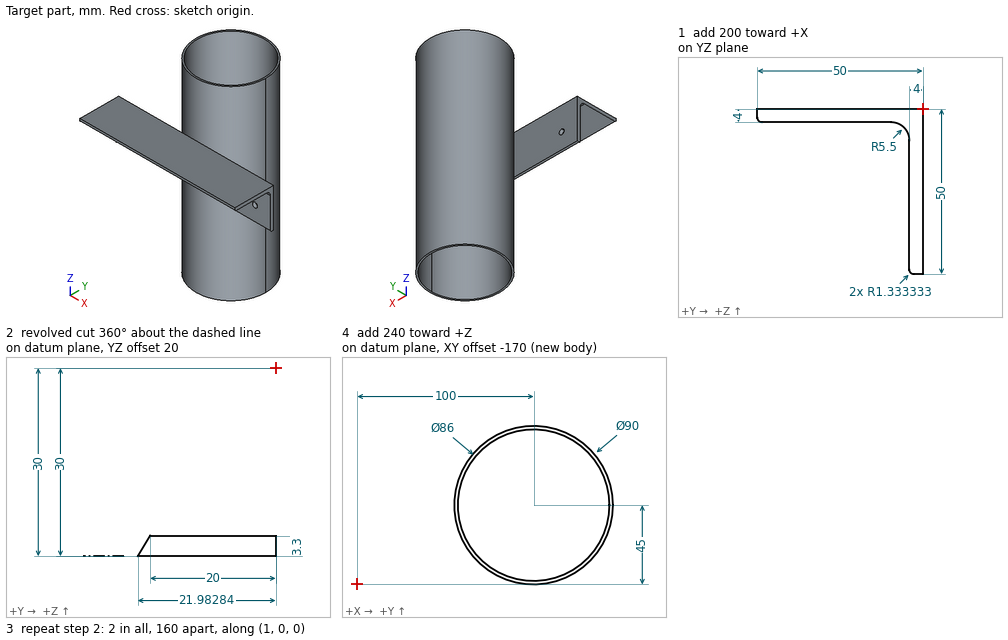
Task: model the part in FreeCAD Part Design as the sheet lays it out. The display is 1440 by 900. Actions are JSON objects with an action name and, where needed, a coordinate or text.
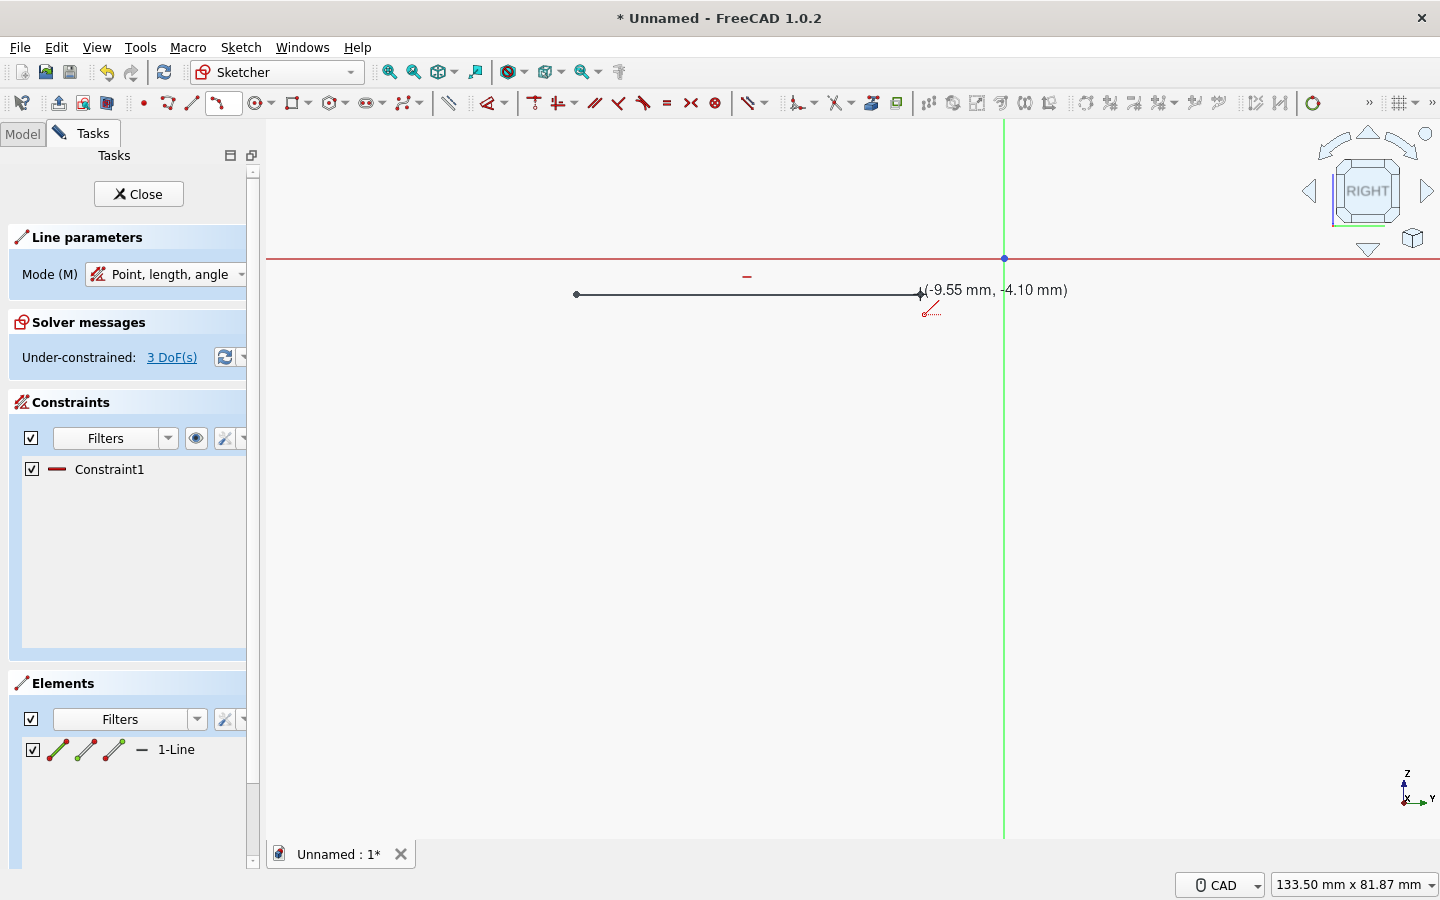
{"action": "left_click", "coordinate": [969, 343]}
{"action": "left_click", "coordinate": [969, 687]}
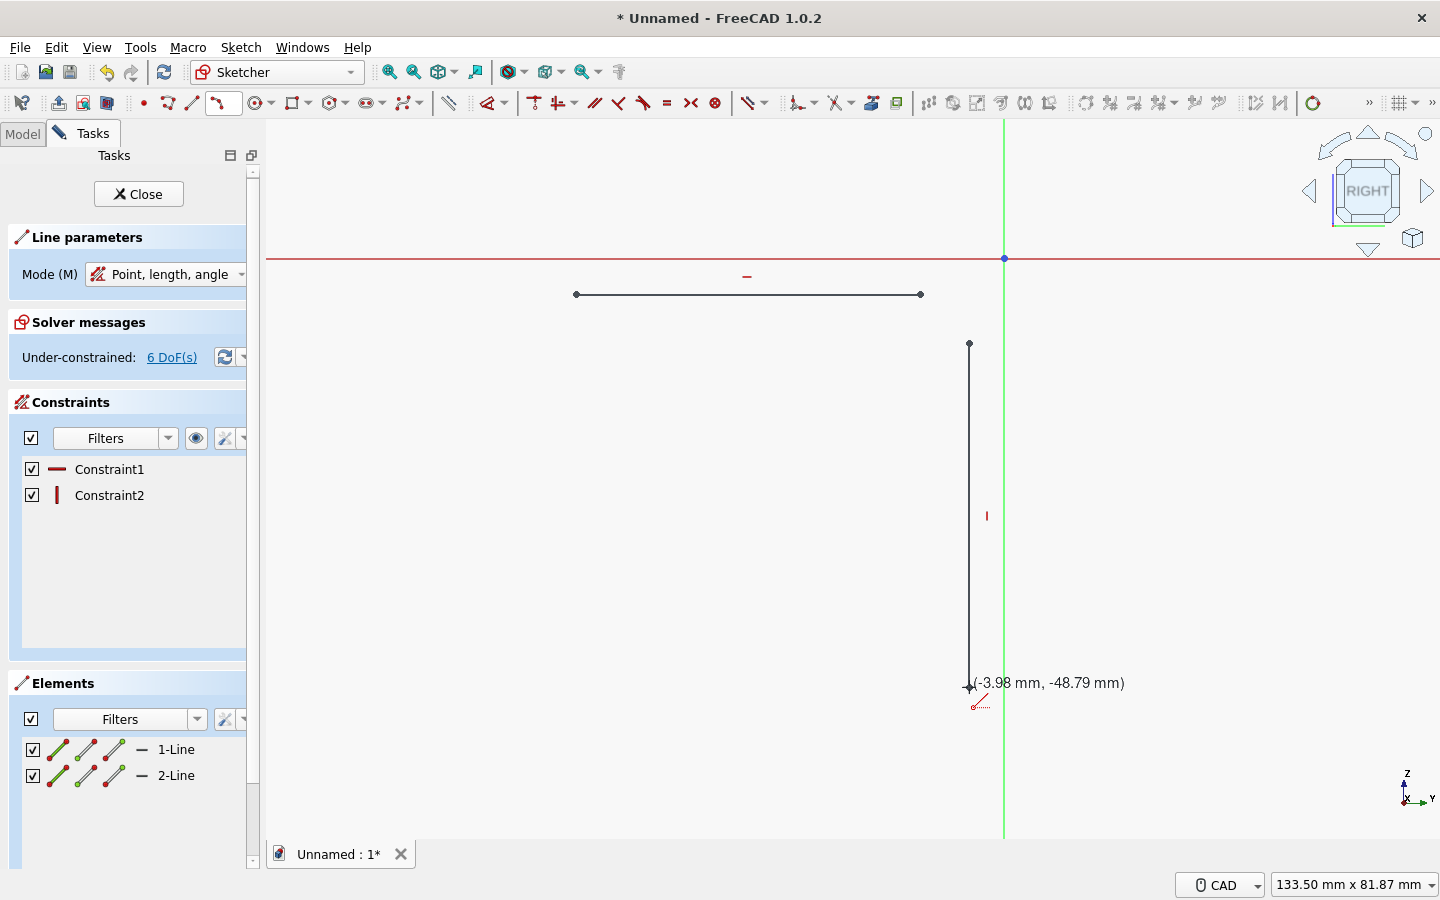
{"action": "left_click", "coordinate": [168, 104]}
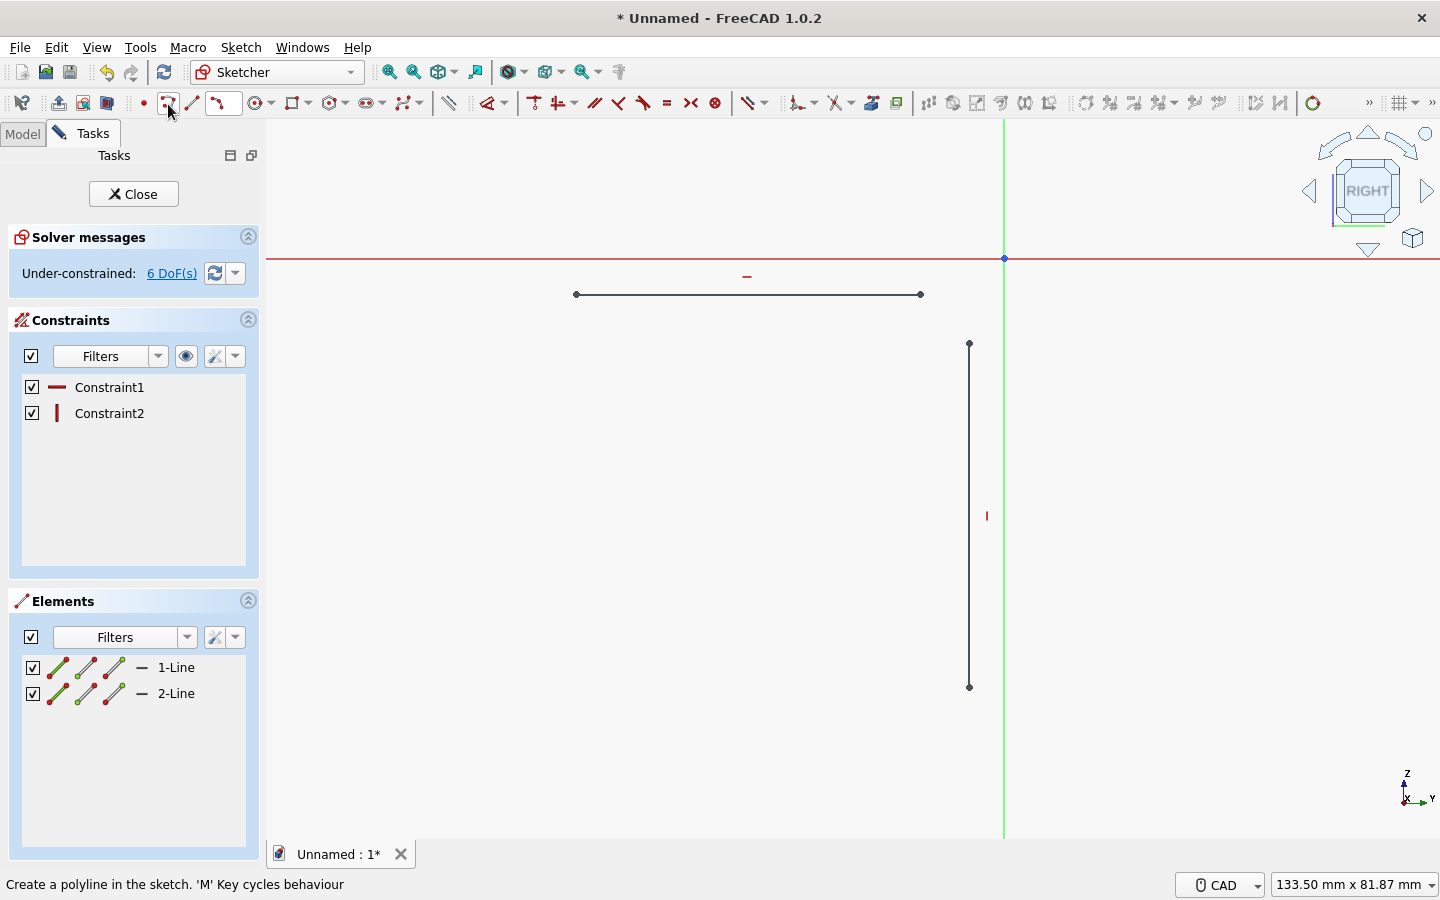
{"action": "left_click", "coordinate": [981, 699]}
{"action": "left_click", "coordinate": [1004, 699]}
{"action": "left_click", "coordinate": [1004, 259]}
{"action": "left_click", "coordinate": [564, 268]}
{"action": "left_click", "coordinate": [564, 282]}
{"action": "right_click", "coordinate": [564, 282]}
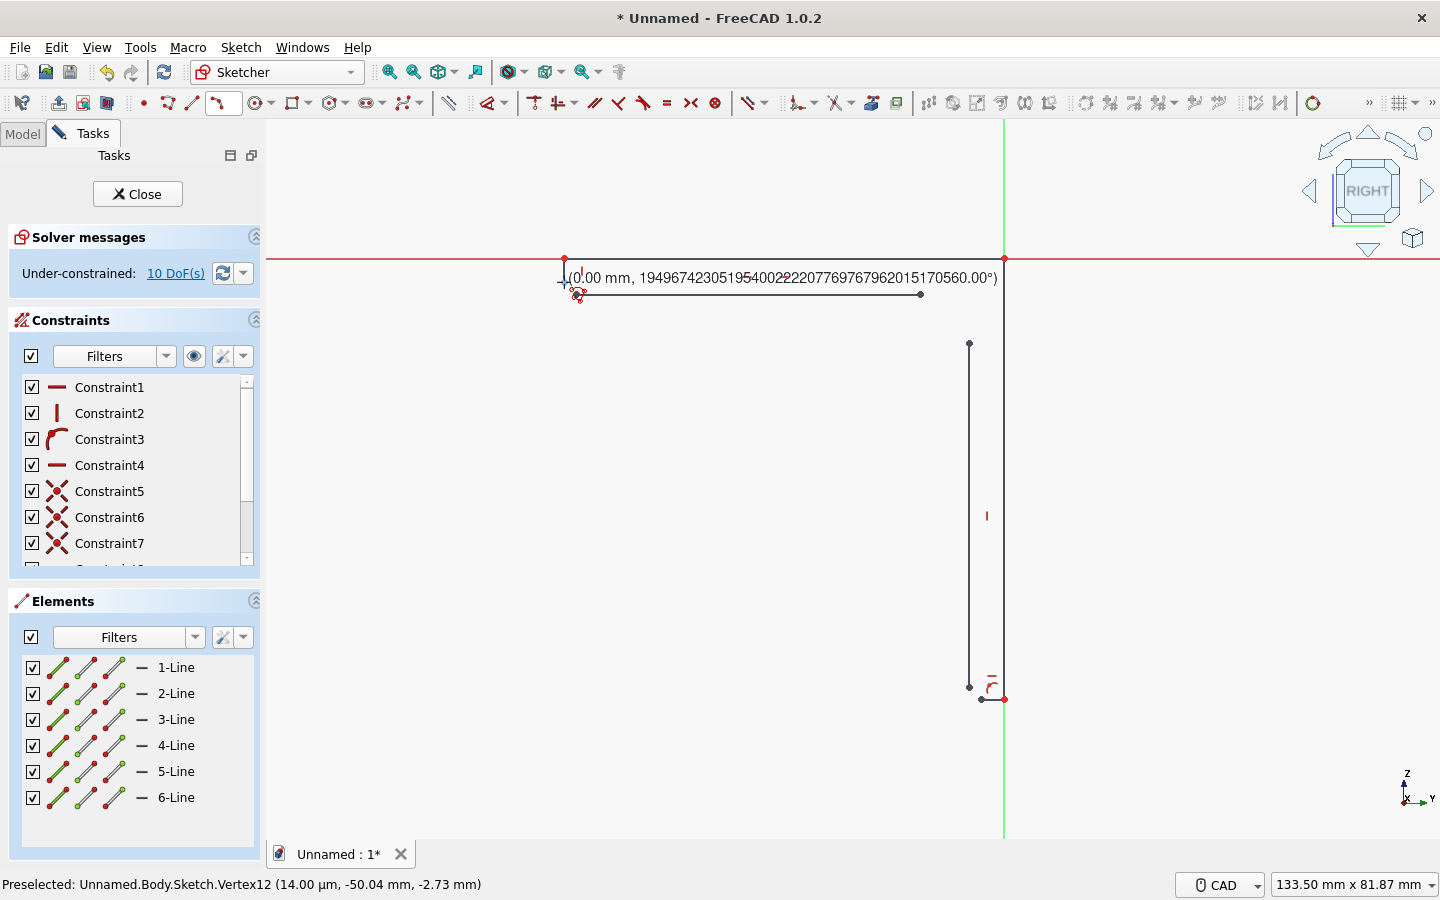
{"action": "left_click", "coordinate": [218, 104]}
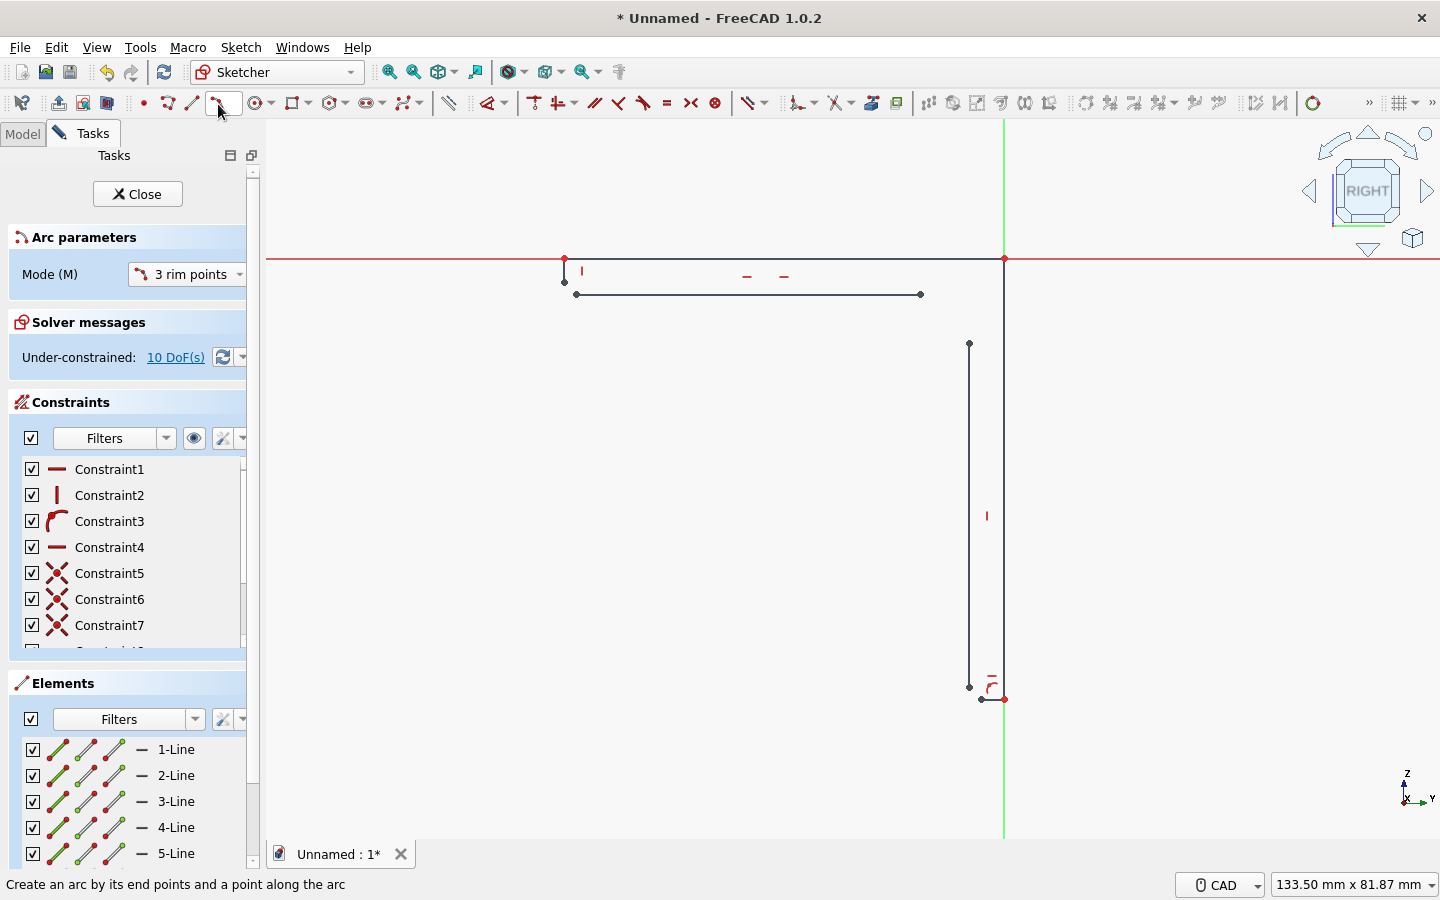
{"action": "left_click", "coordinate": [920, 295]}
{"action": "left_click", "coordinate": [969, 344]}
{"action": "left_click", "coordinate": [955, 308]}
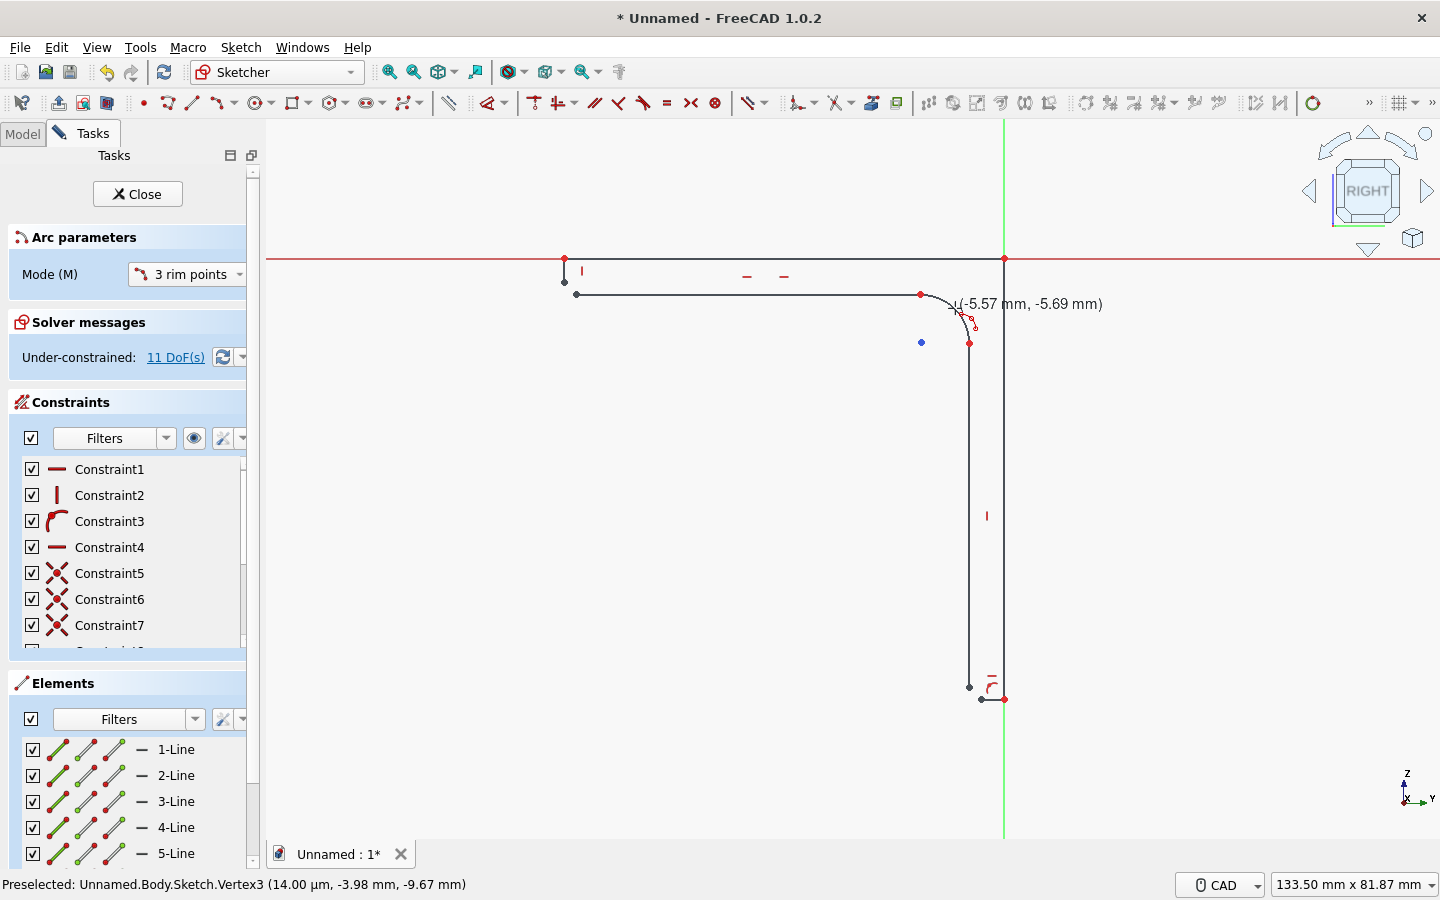
{"action": "left_click", "coordinate": [969, 688]}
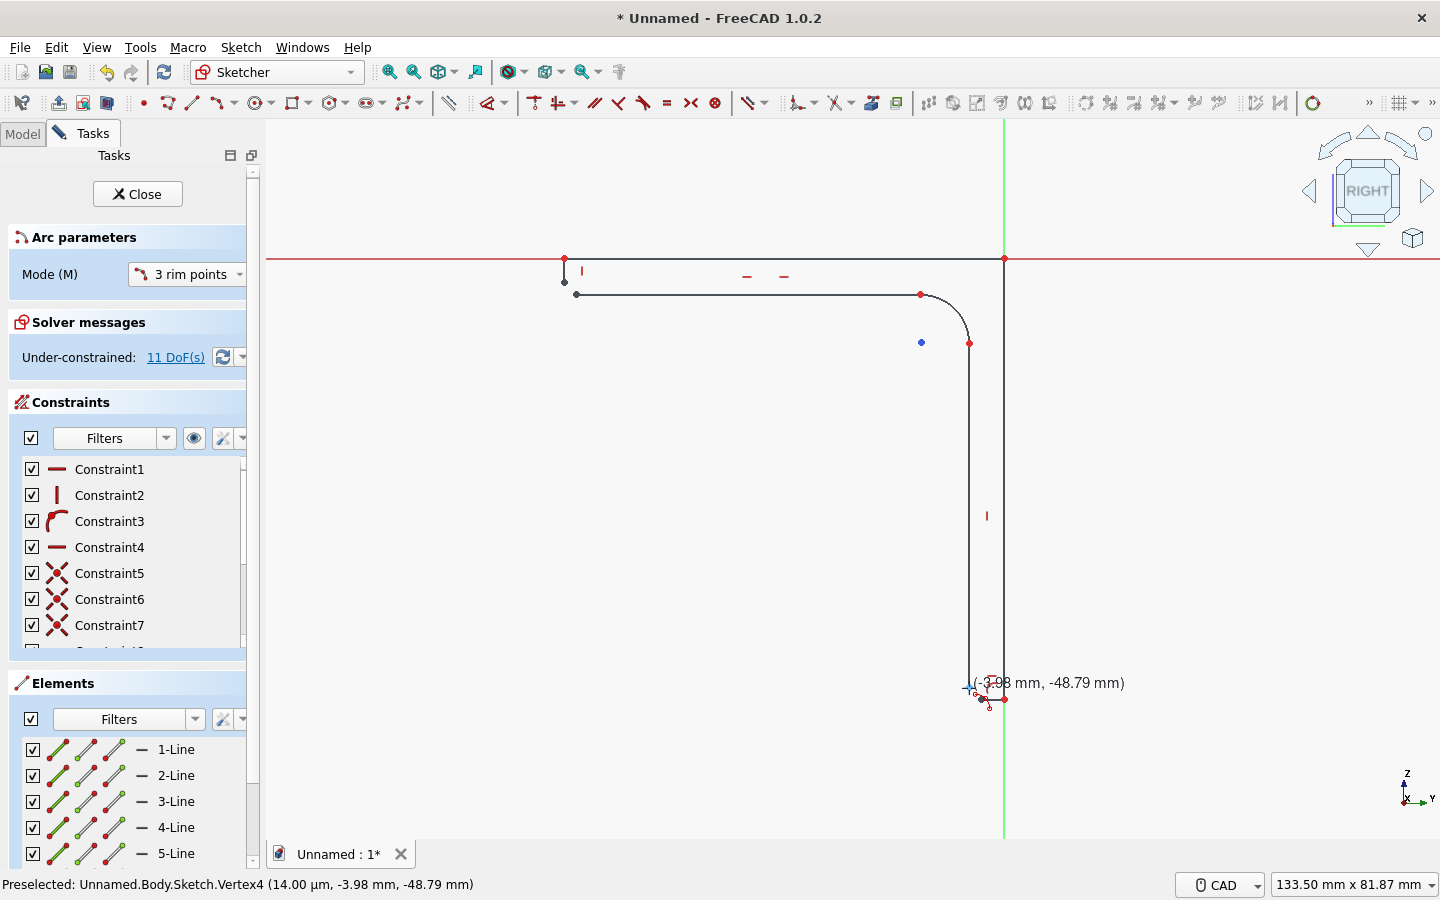
{"action": "scroll", "coordinate": [981, 699], "scroll_direction": "up", "scroll_amount": 2}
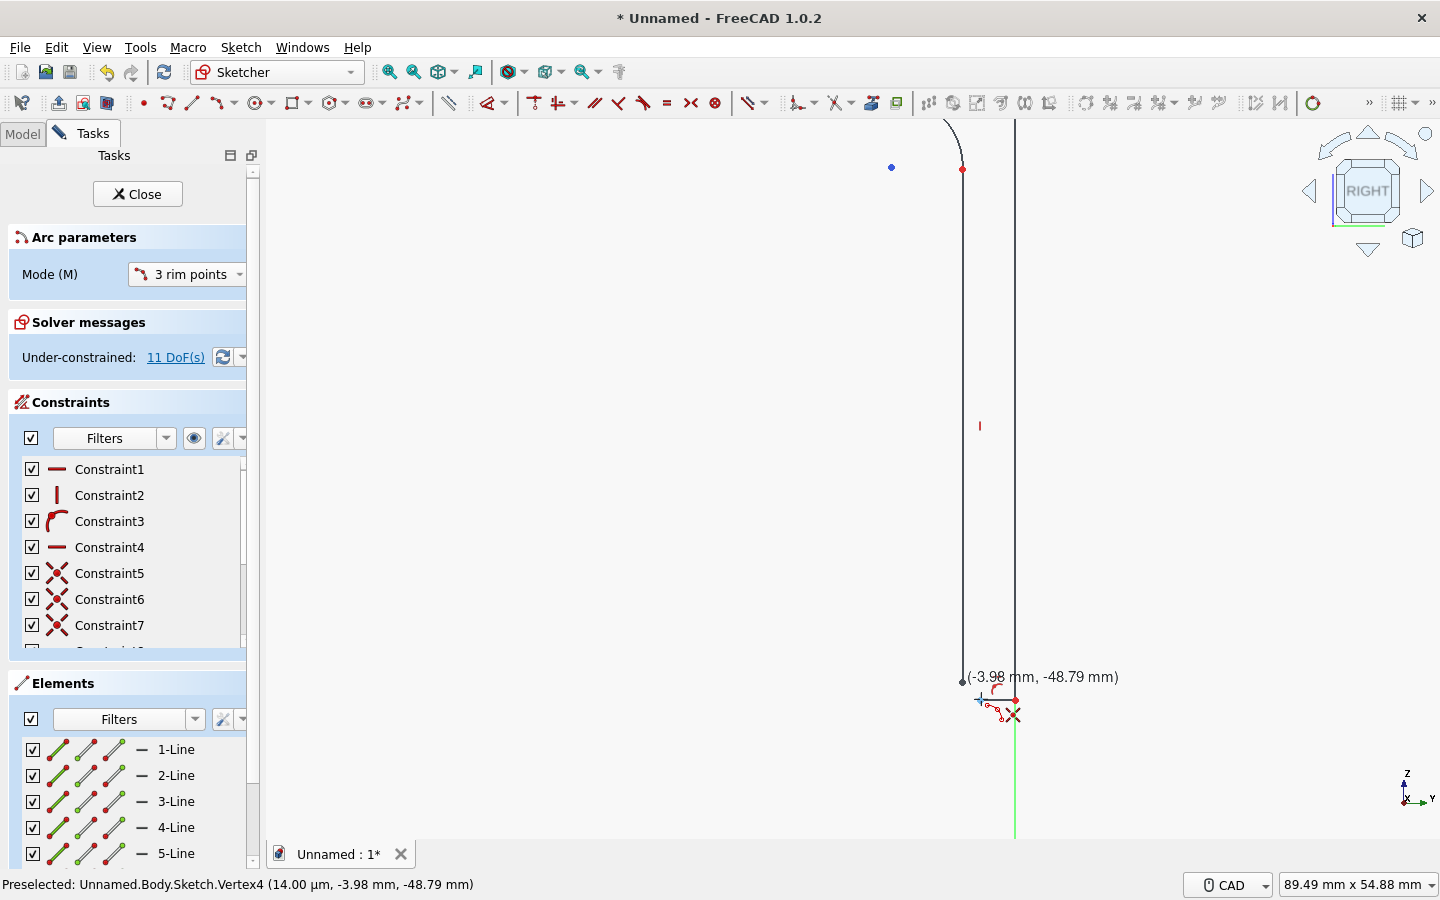
{"action": "left_click", "coordinate": [981, 700]}